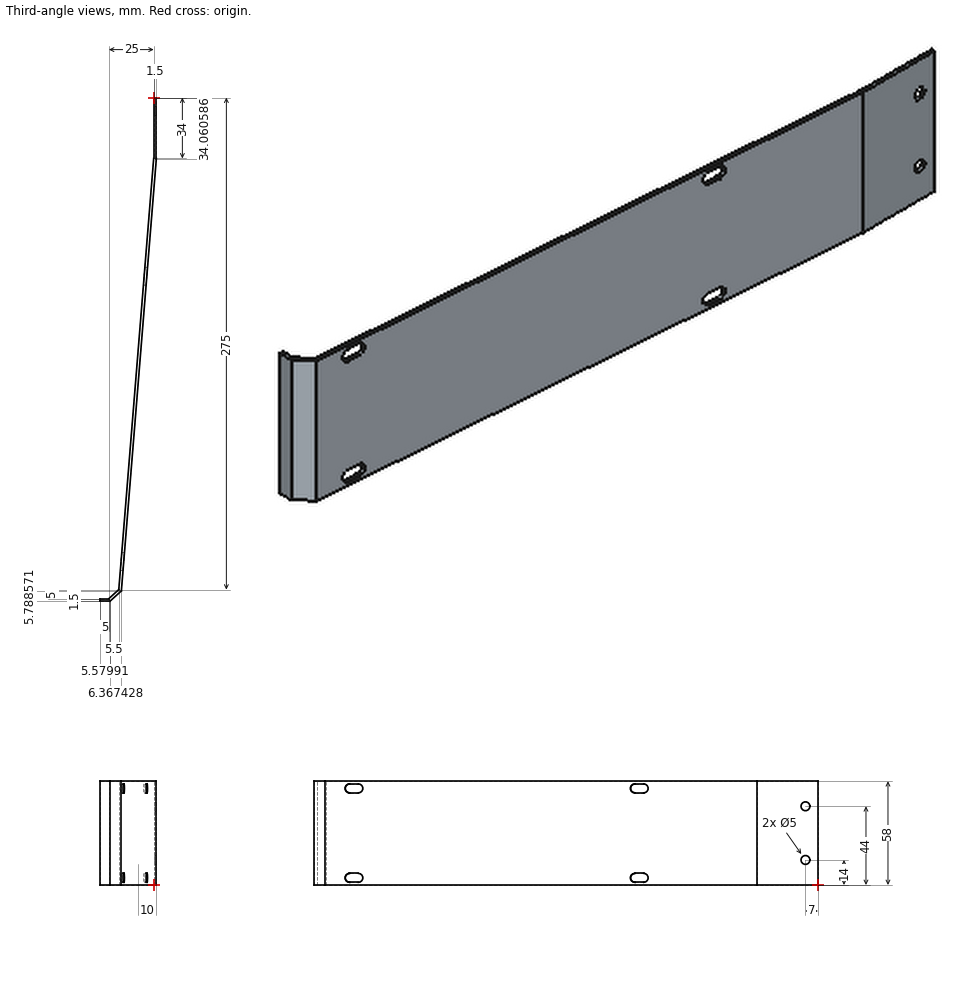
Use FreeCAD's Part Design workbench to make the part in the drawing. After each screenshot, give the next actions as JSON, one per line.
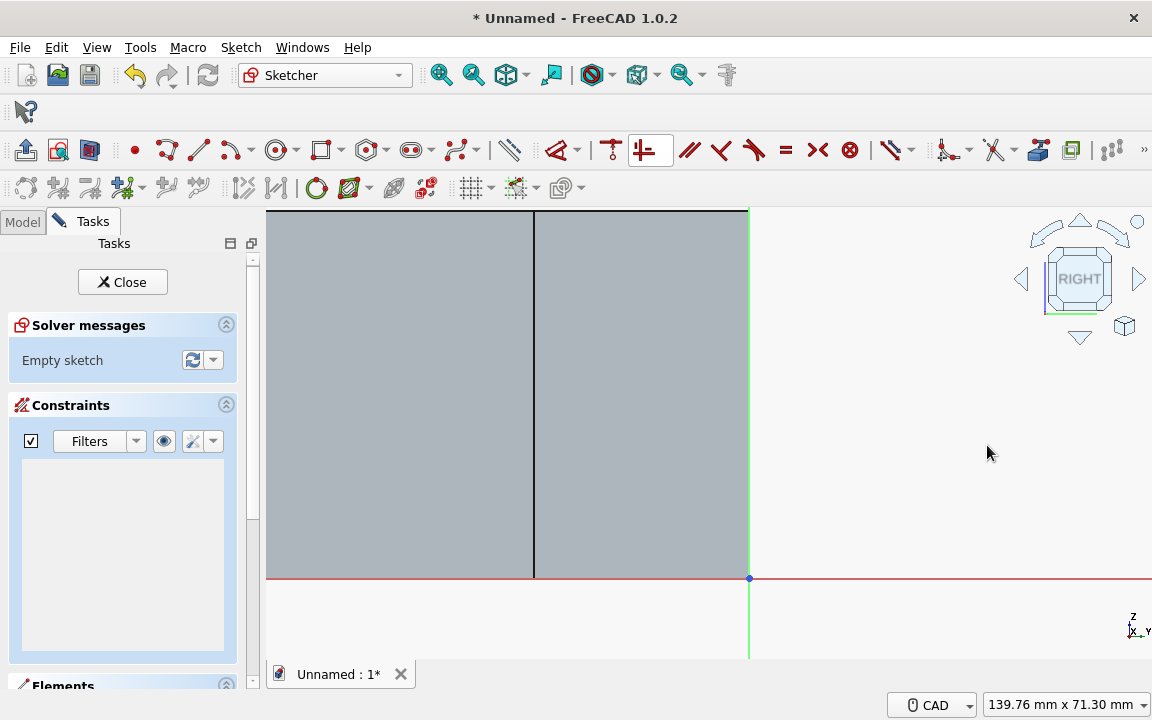
{"action": "left_click", "coordinate": [276, 150]}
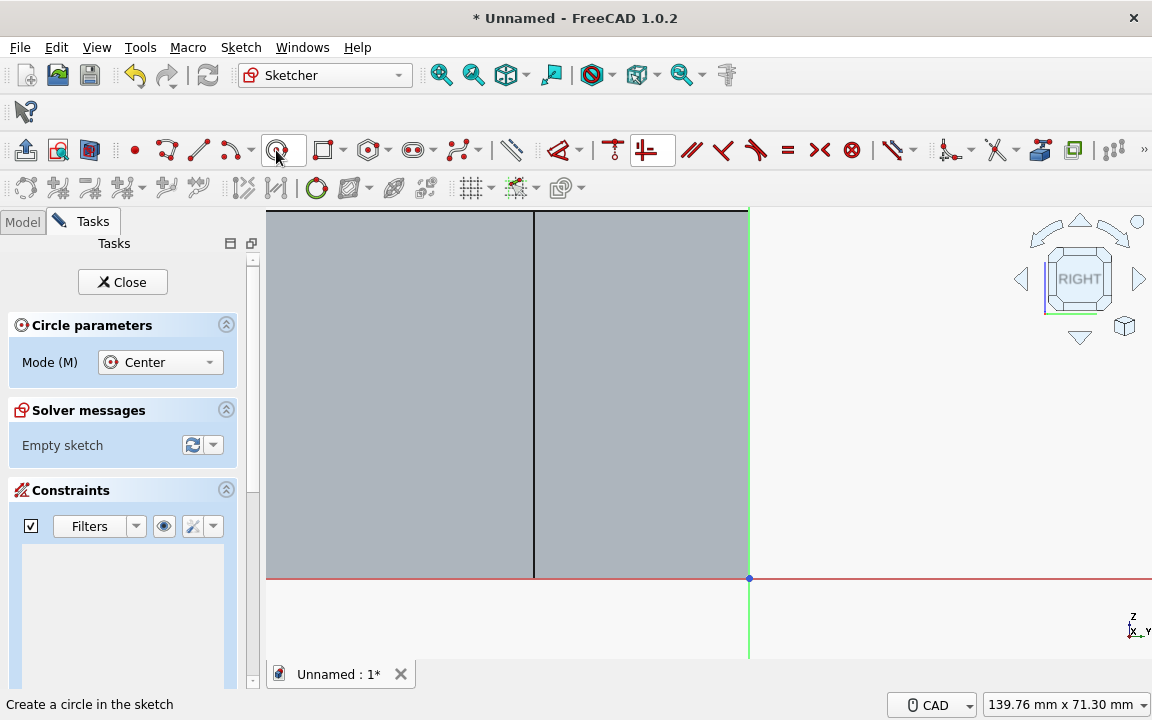
{"action": "scroll", "coordinate": [705, 490], "scroll_direction": "up", "scroll_amount": 2}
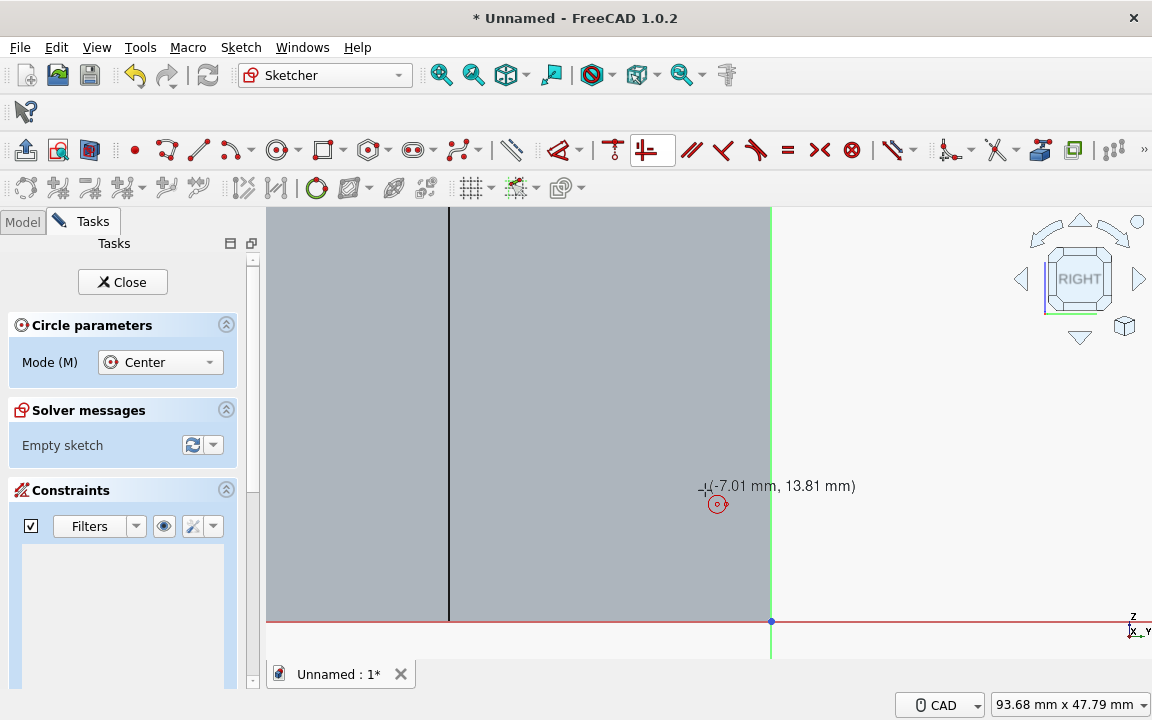
{"action": "left_click", "coordinate": [705, 489]}
{"action": "left_click", "coordinate": [722, 473]}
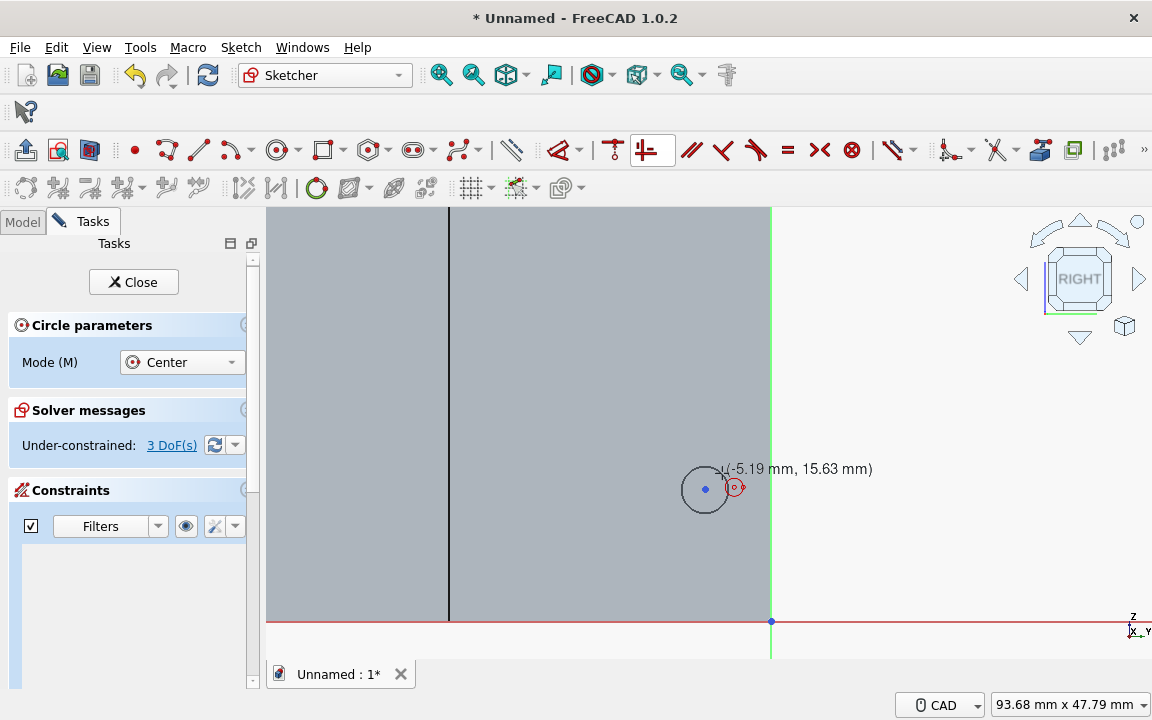
{"action": "scroll", "coordinate": [466, 496], "scroll_direction": "down", "scroll_amount": 2}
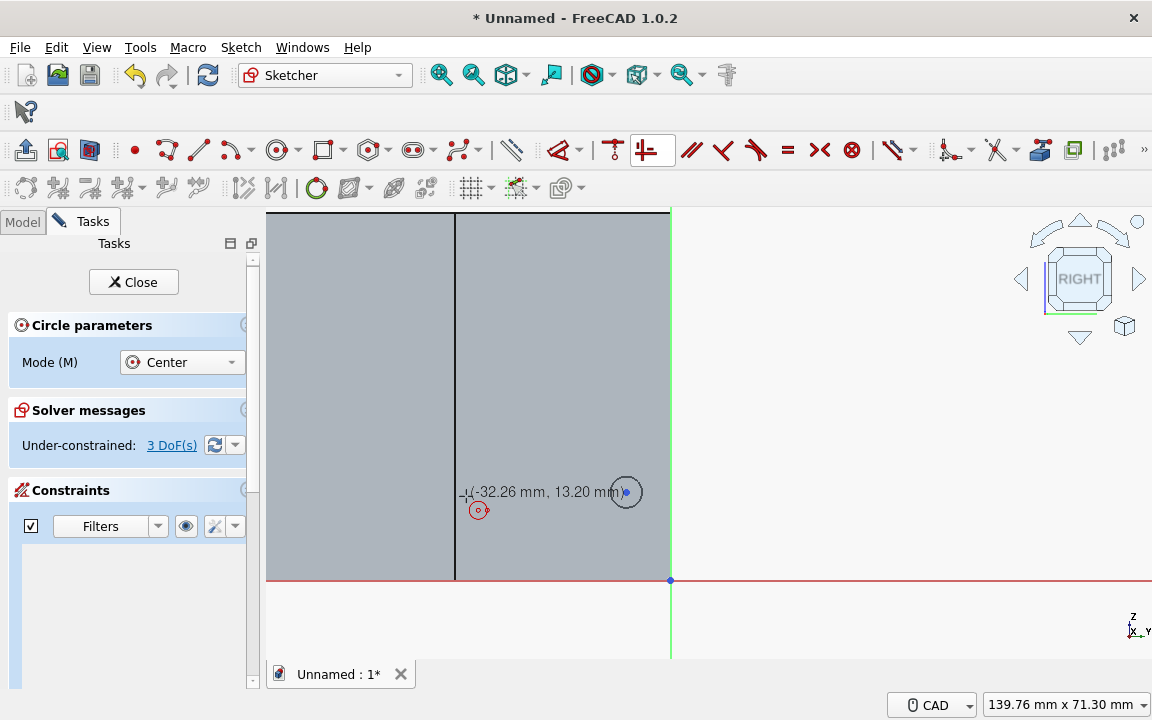
{"action": "scroll", "coordinate": [626, 302], "scroll_direction": "up", "scroll_amount": 2}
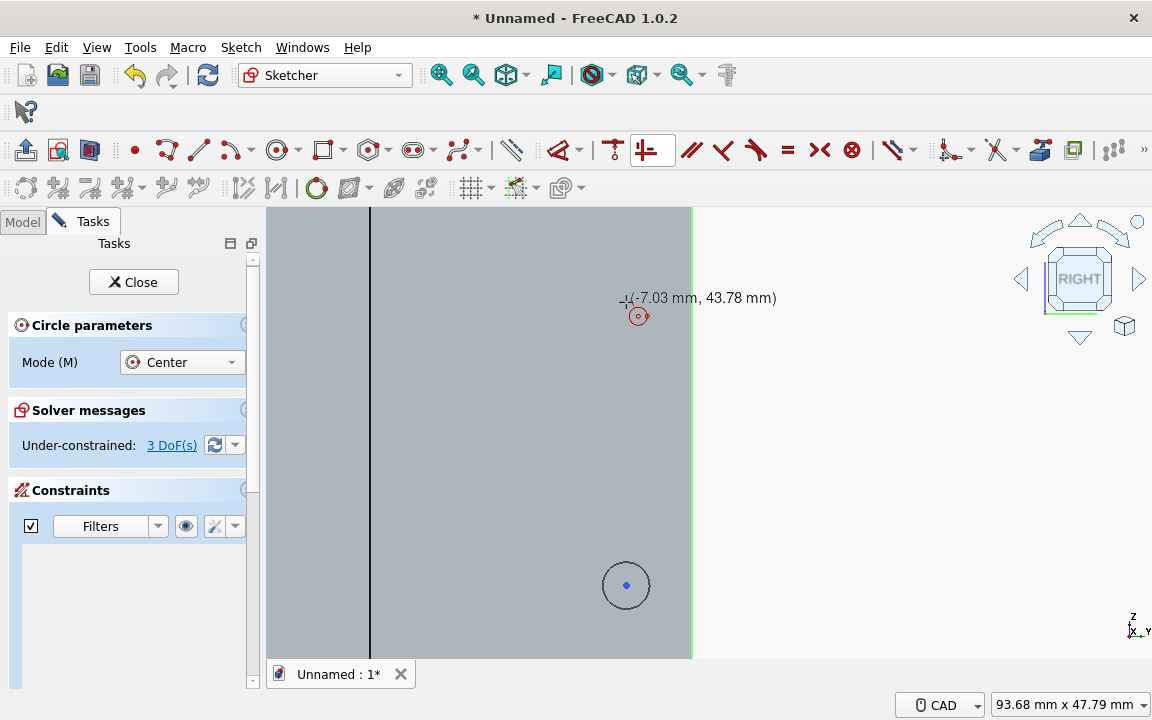
{"action": "left_click", "coordinate": [626, 301]}
{"action": "left_click", "coordinate": [643, 285]}
{"action": "key", "text": "Escape"}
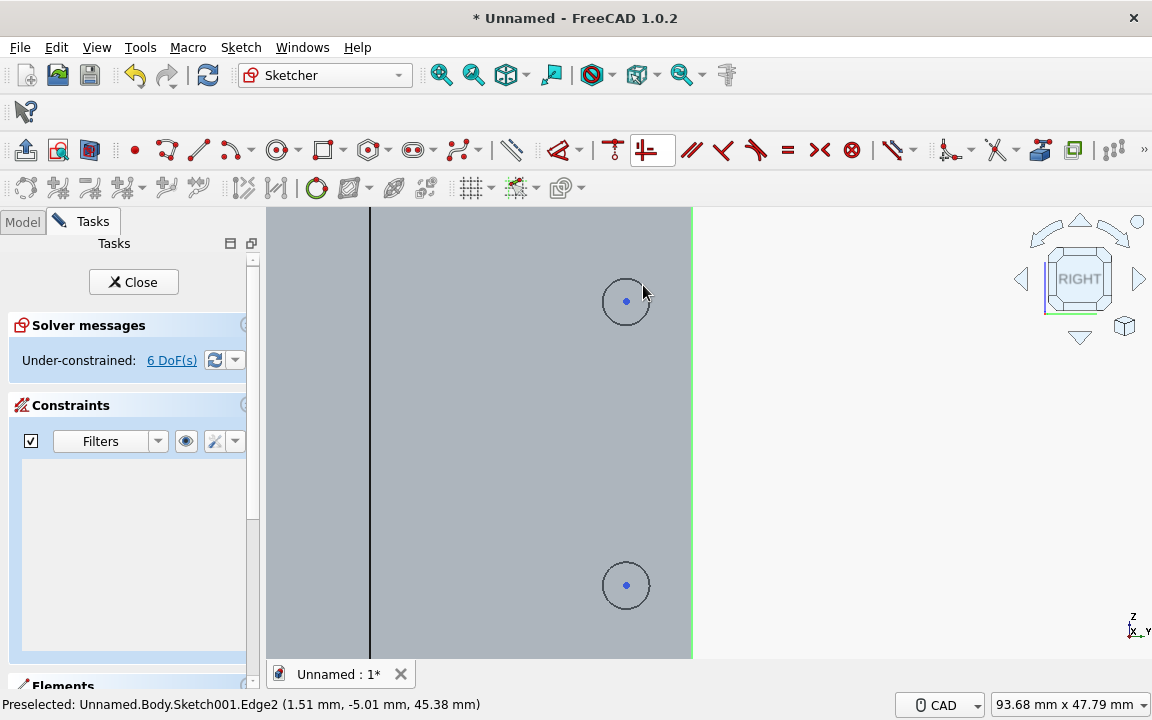
{"action": "left_click", "coordinate": [643, 569]}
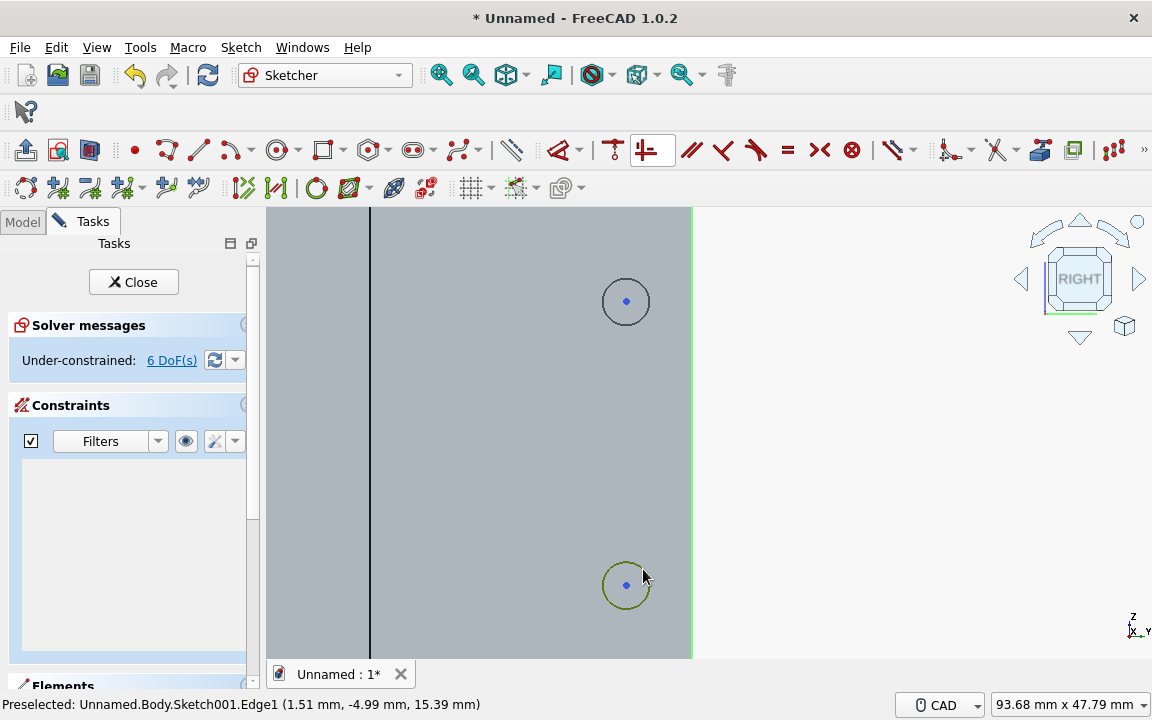
{"action": "left_click", "coordinate": [642, 285]}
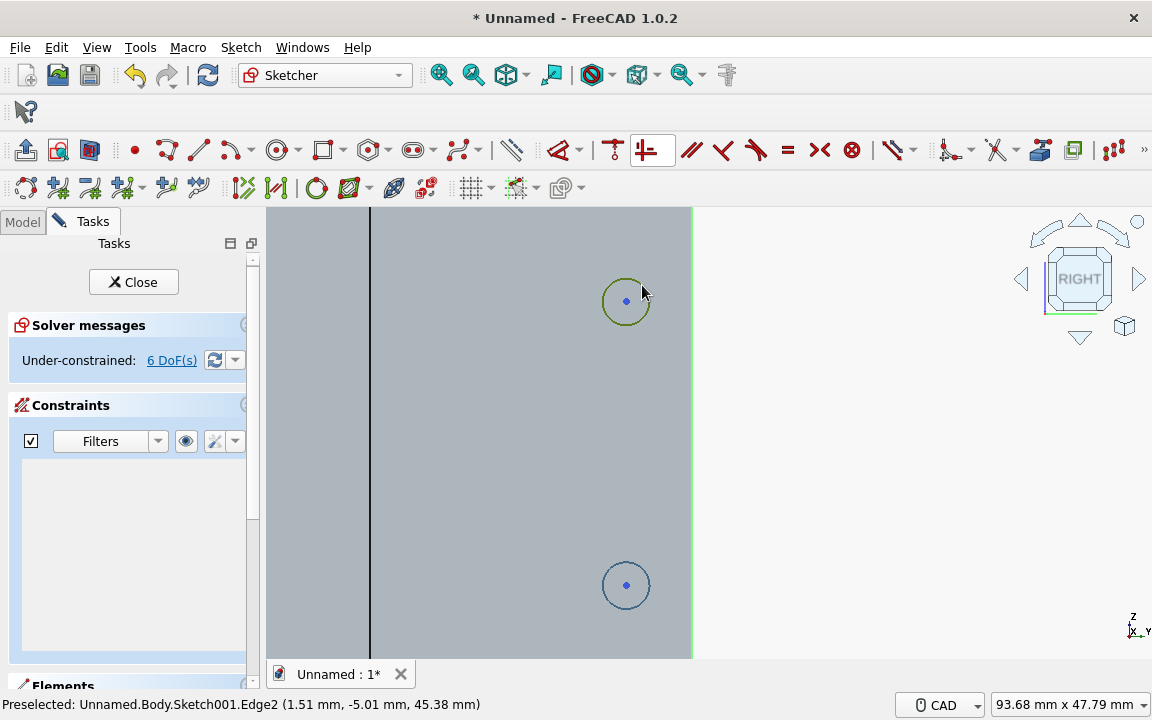
{"action": "left_click", "coordinate": [788, 150]}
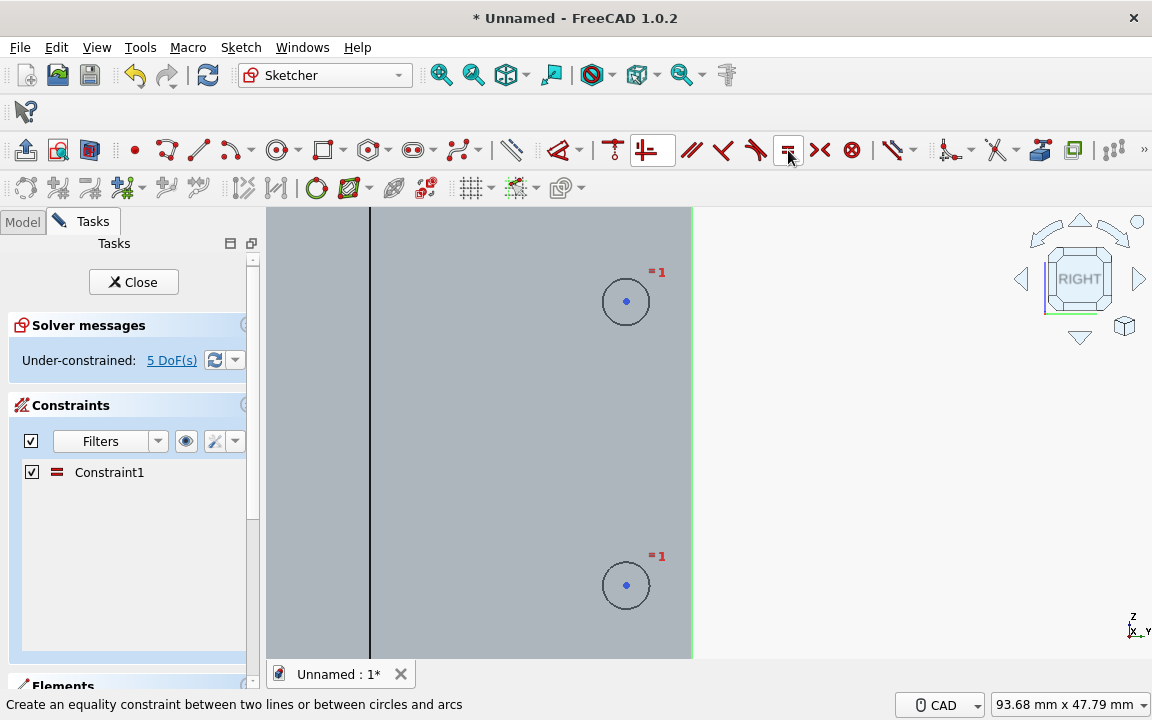
{"action": "left_click", "coordinate": [626, 586]}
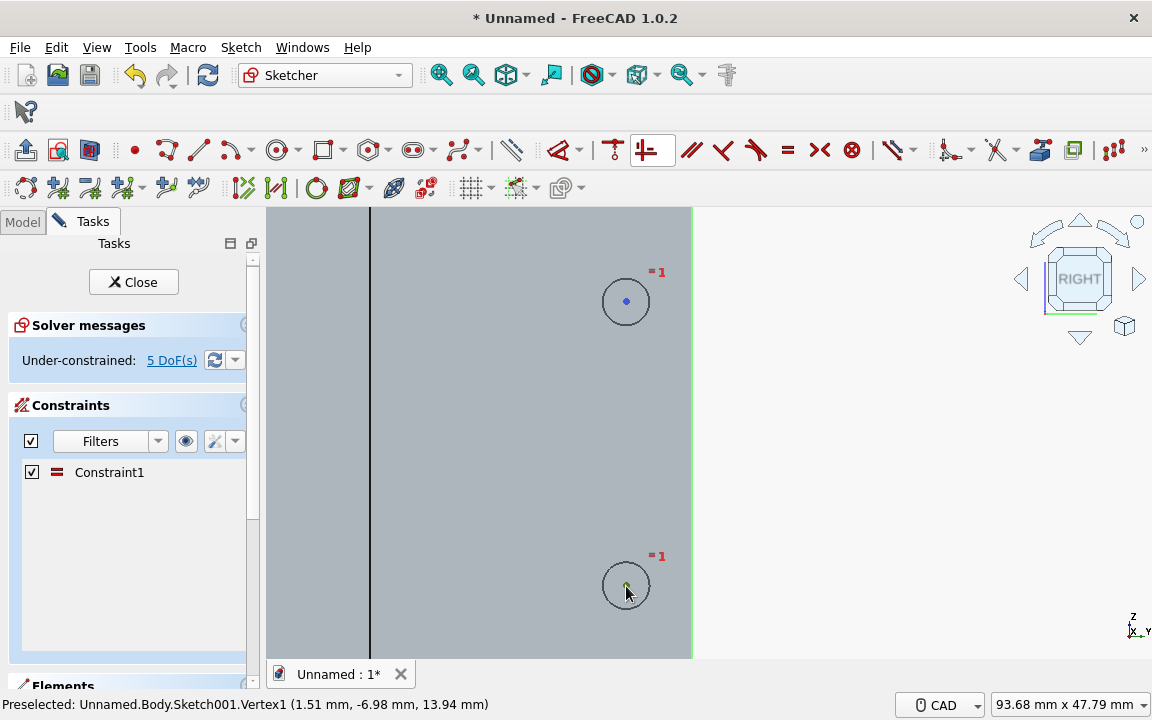
{"action": "left_click", "coordinate": [626, 302]}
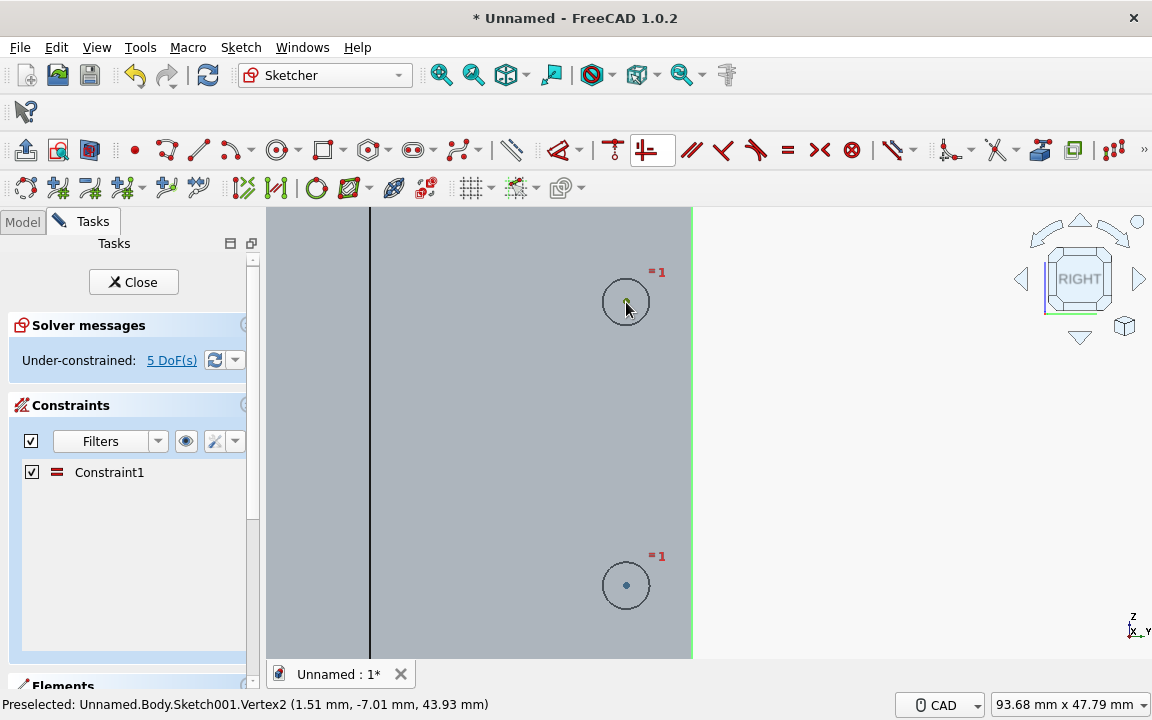
{"action": "left_click", "coordinate": [670, 150]}